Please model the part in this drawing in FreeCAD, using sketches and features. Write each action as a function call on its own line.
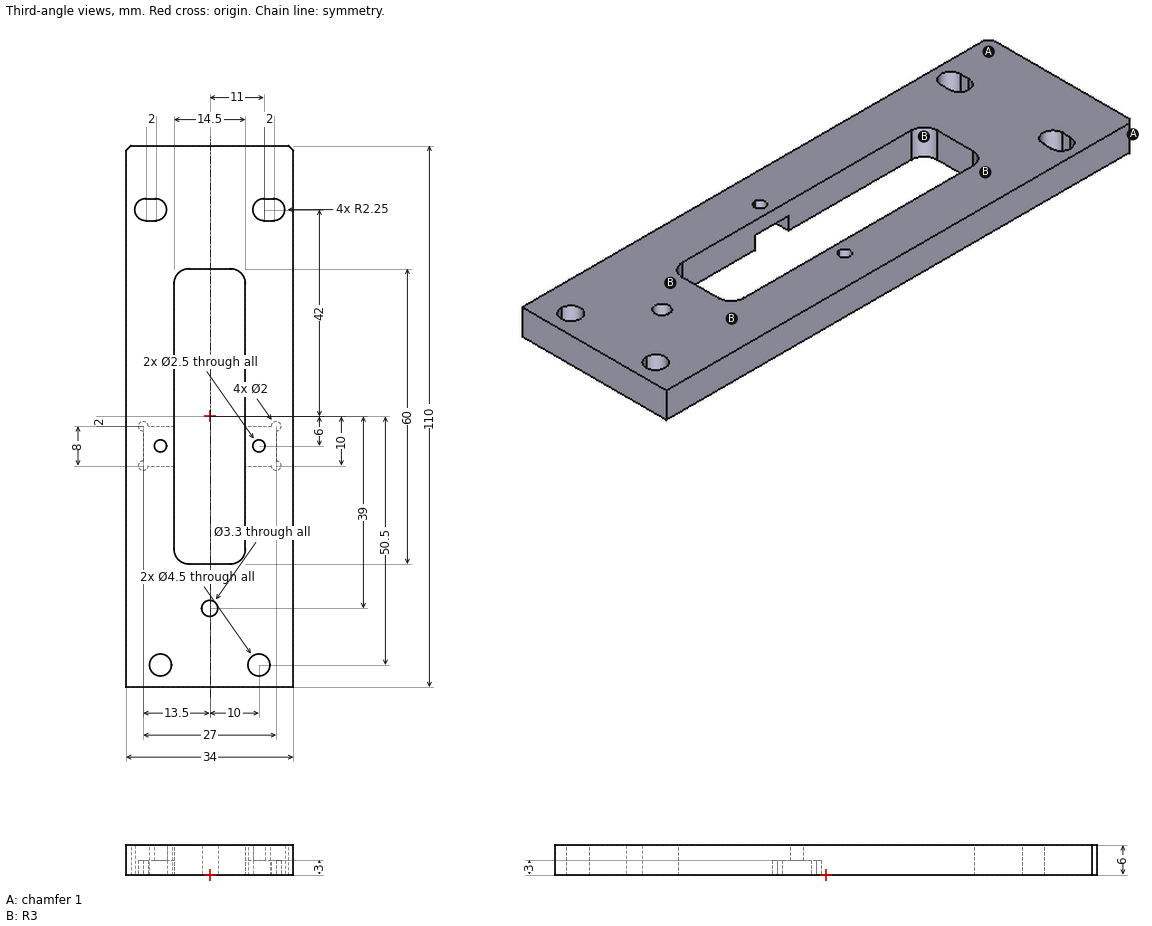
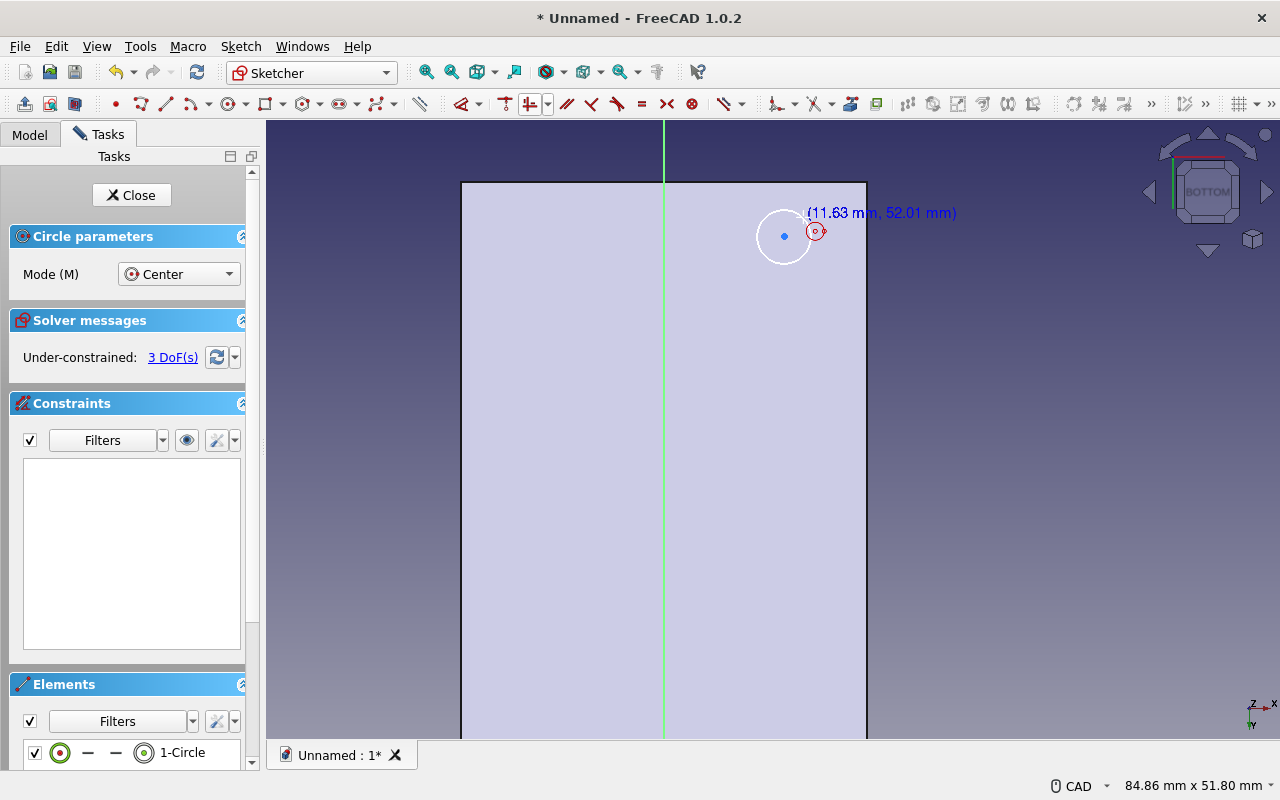
click(545, 236)
click(564, 217)
key(Escape)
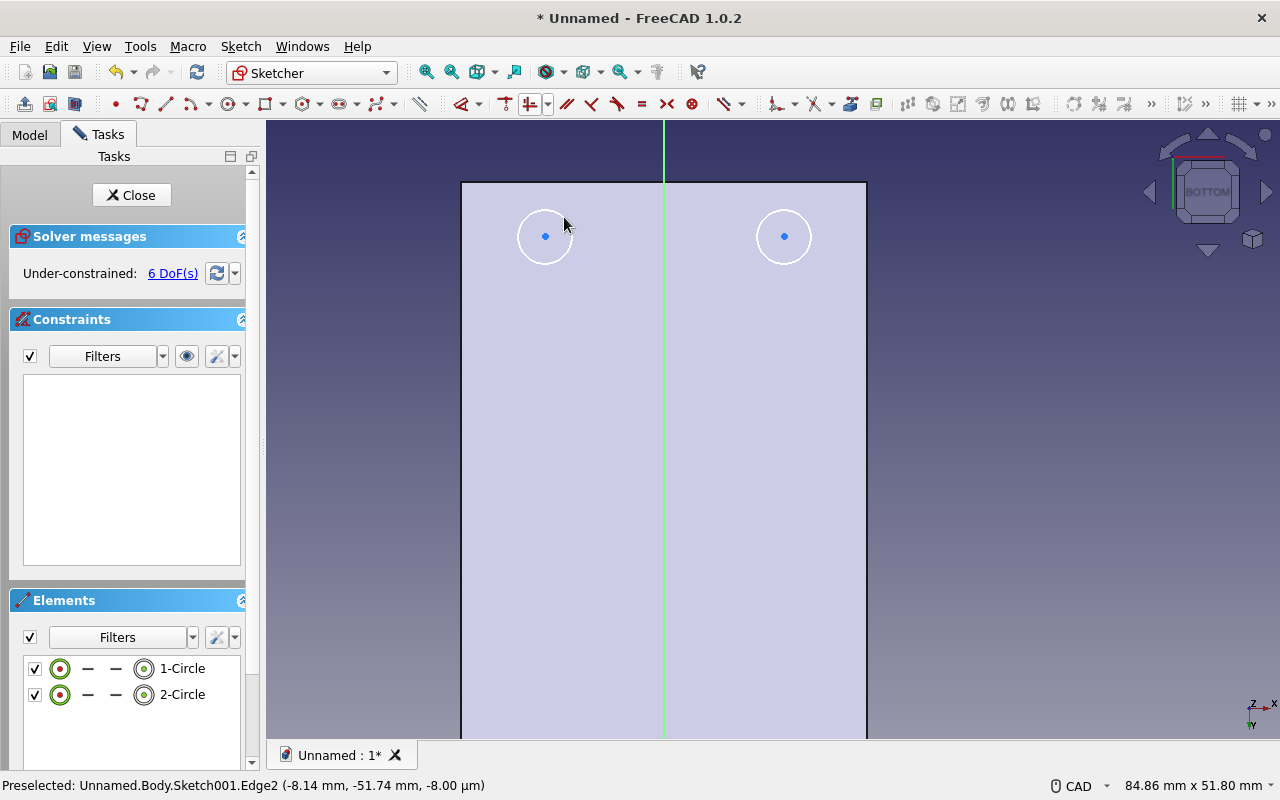
click(803, 218)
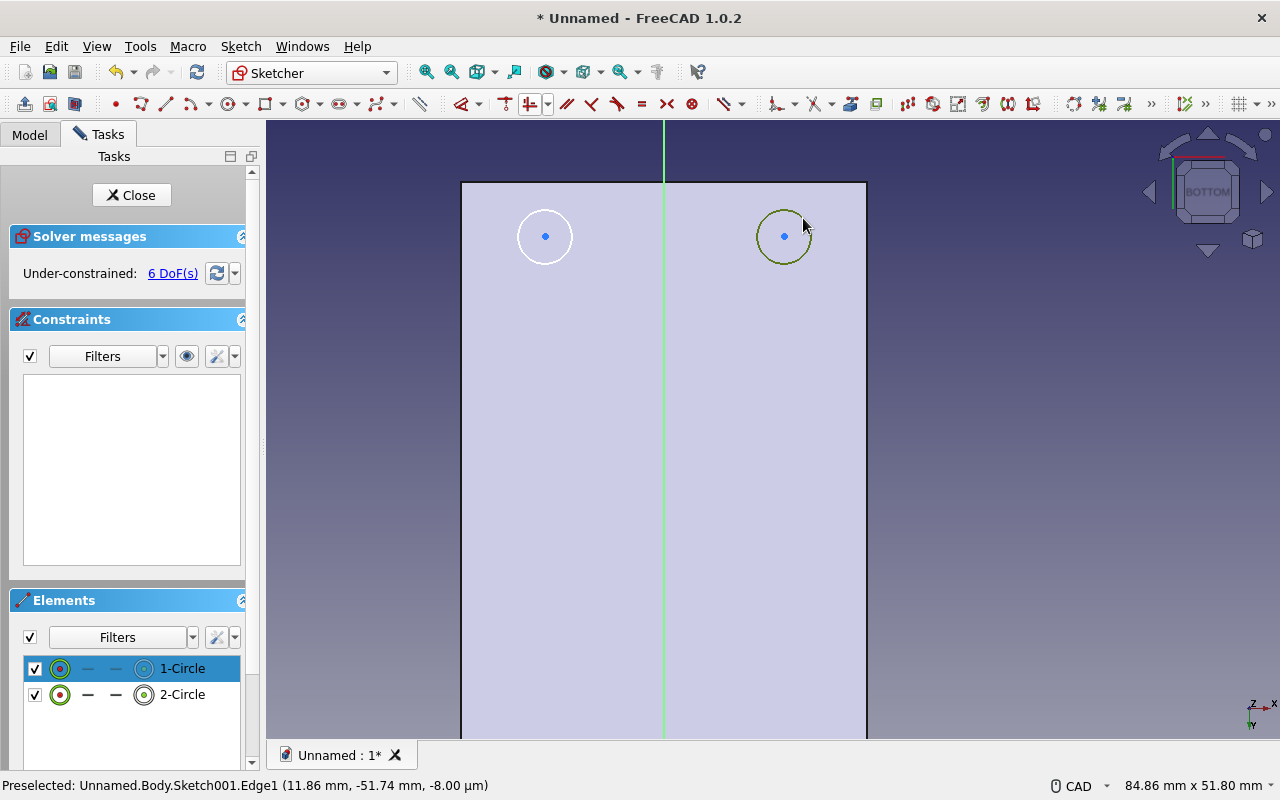
click(564, 218)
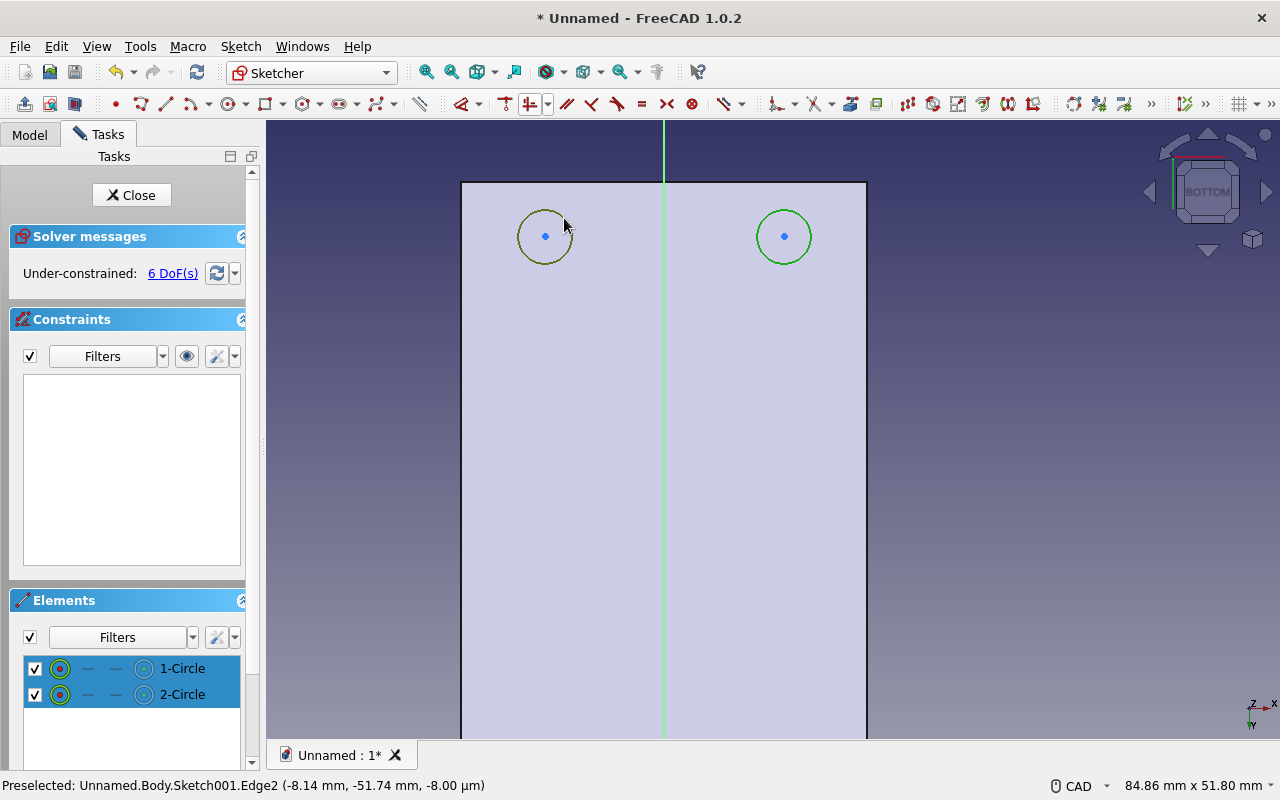
key(e)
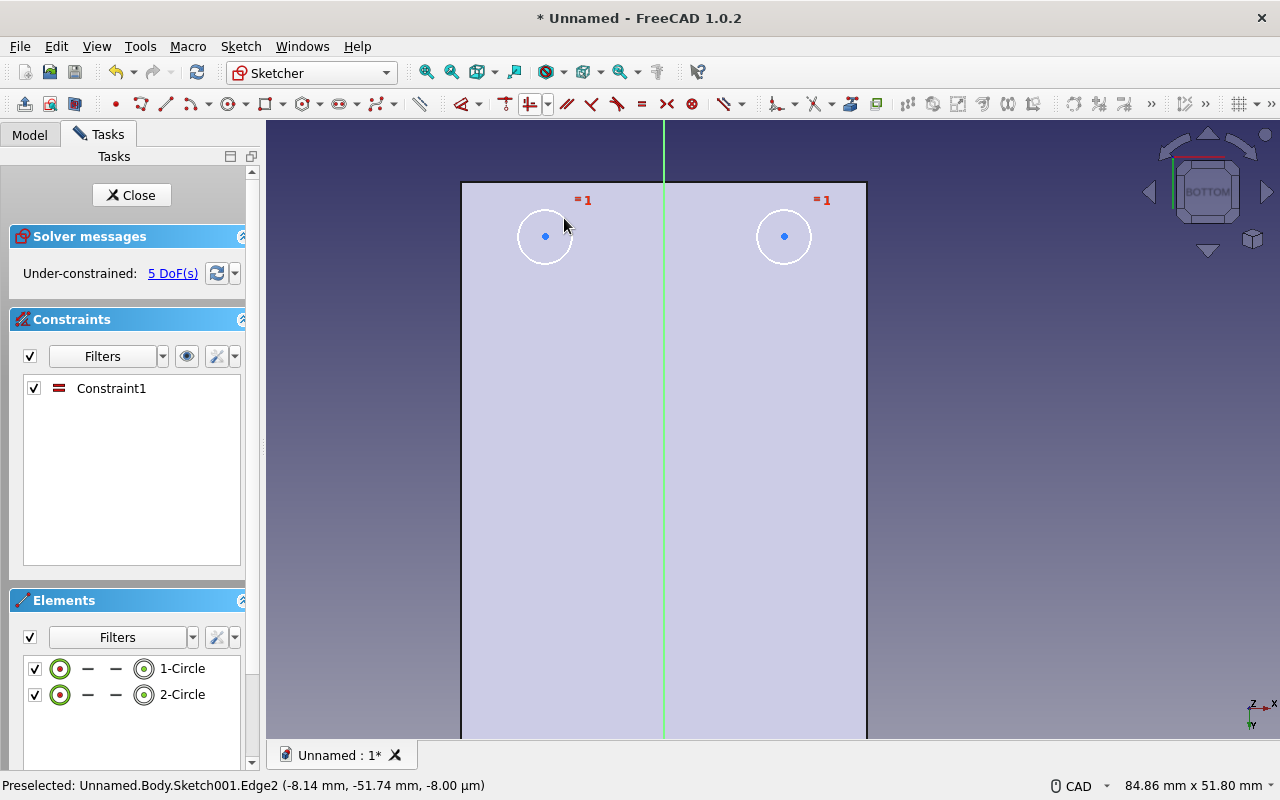
click(784, 237)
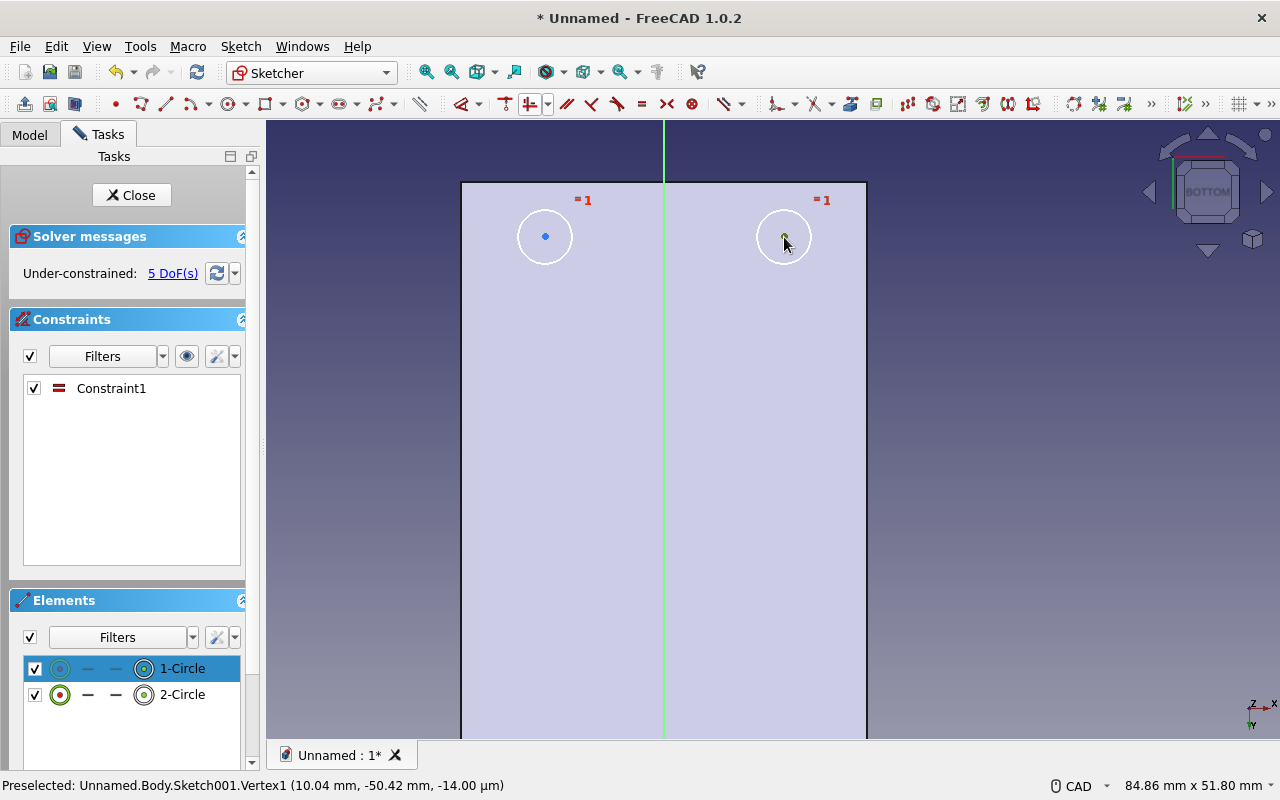
click(545, 237)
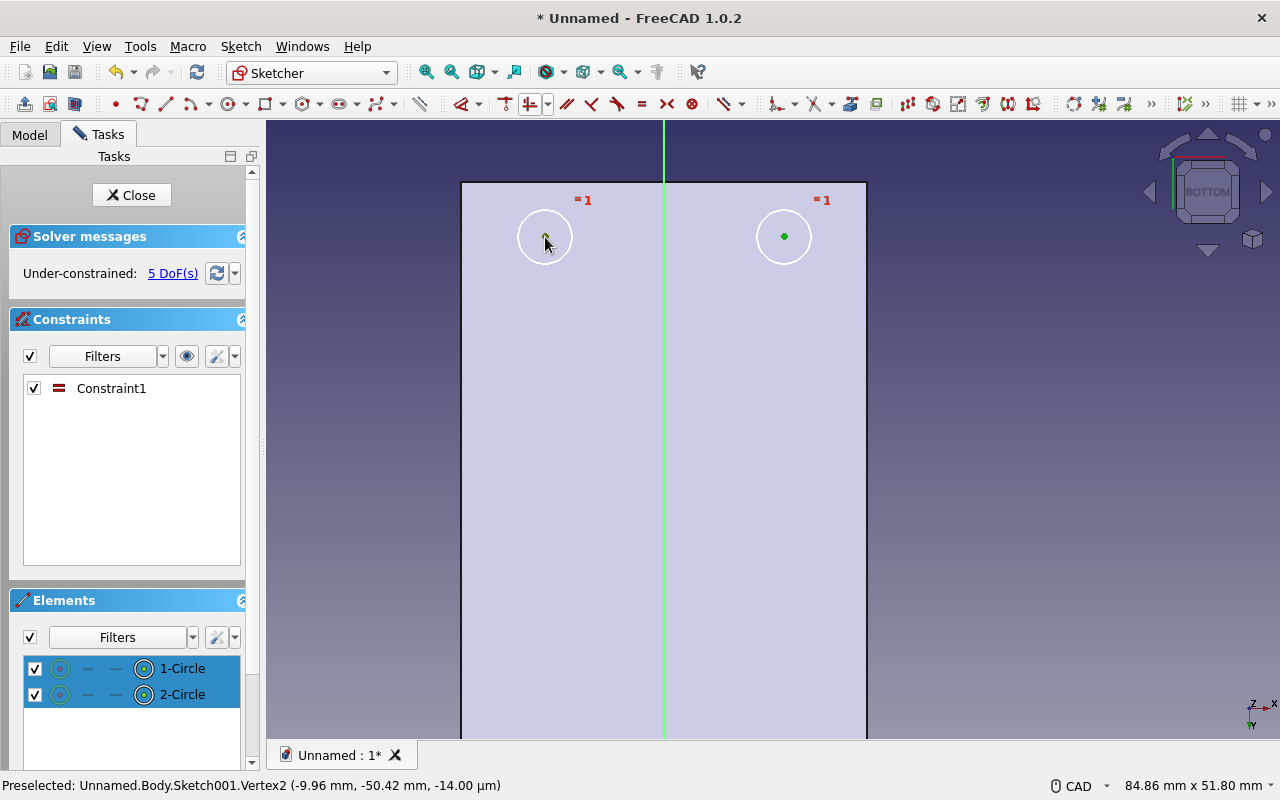
click(664, 671)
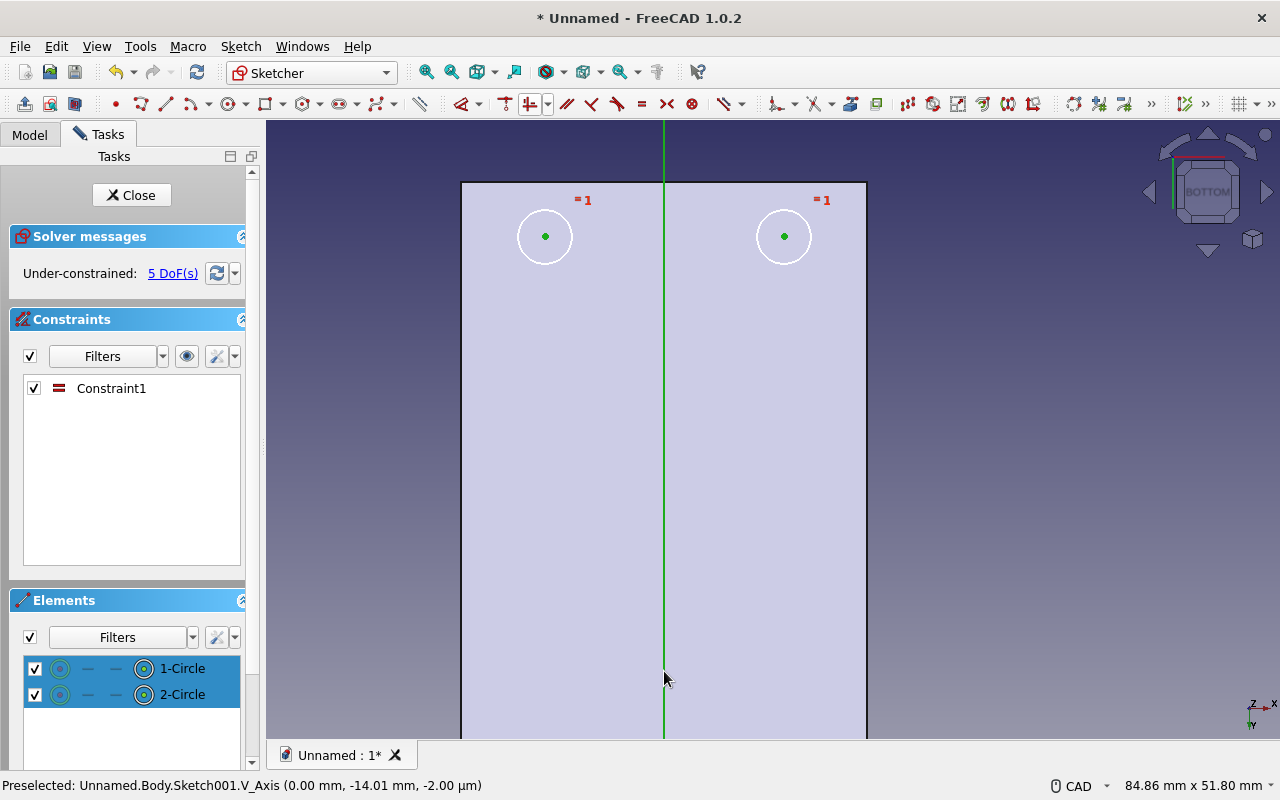
key(s)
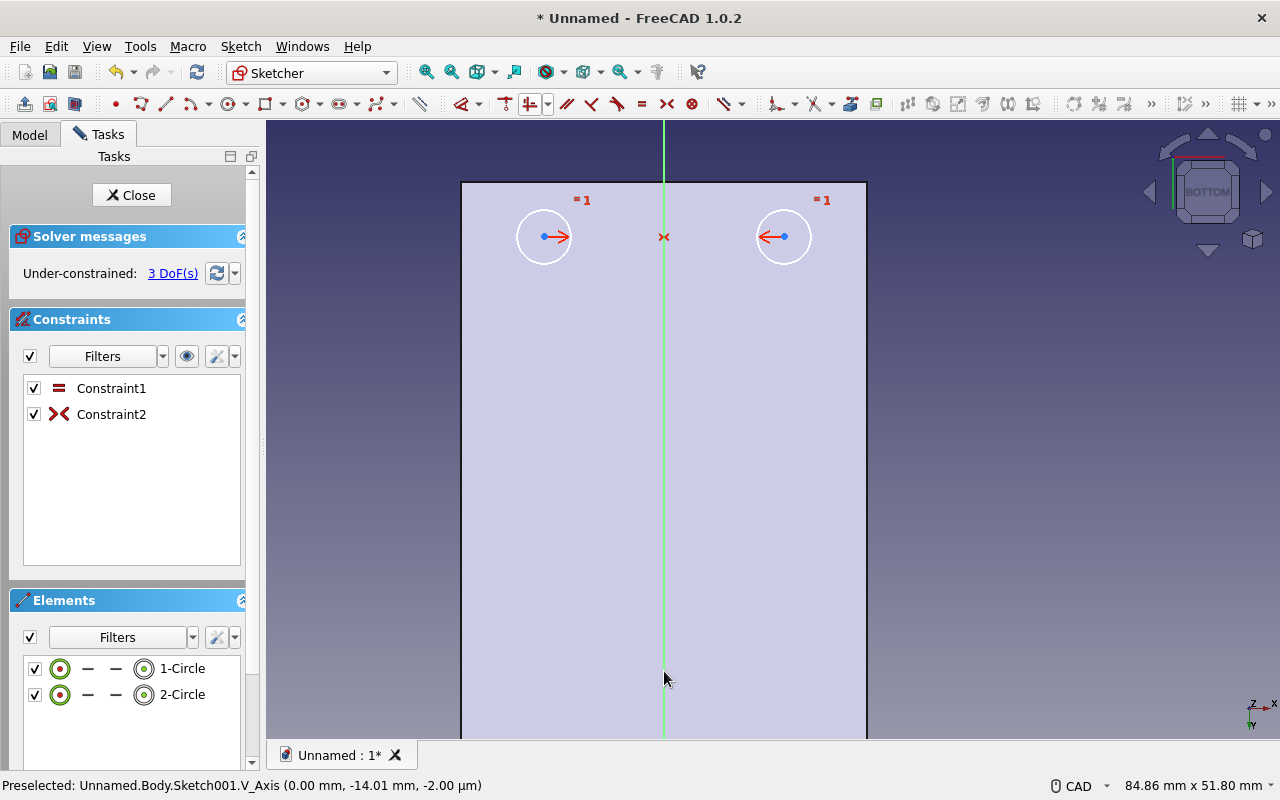
click(803, 218)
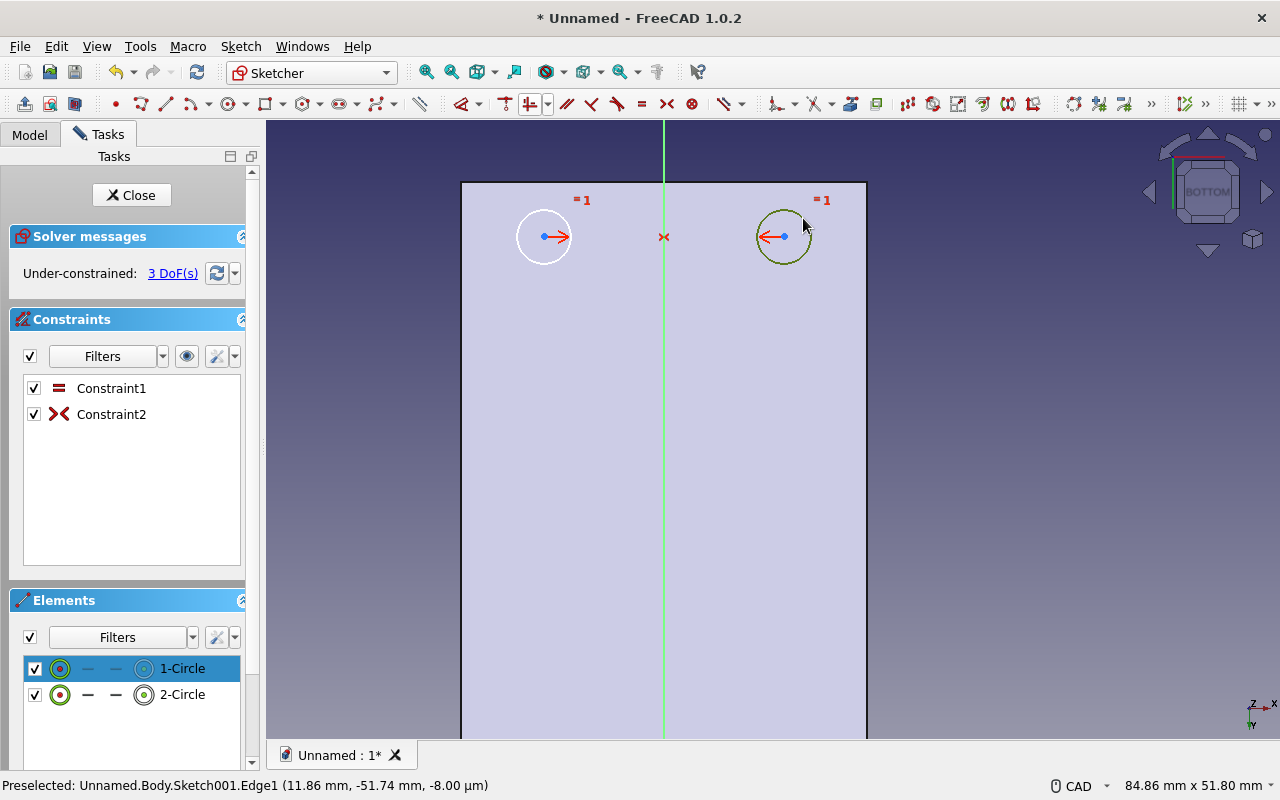
key(k)
key(o)